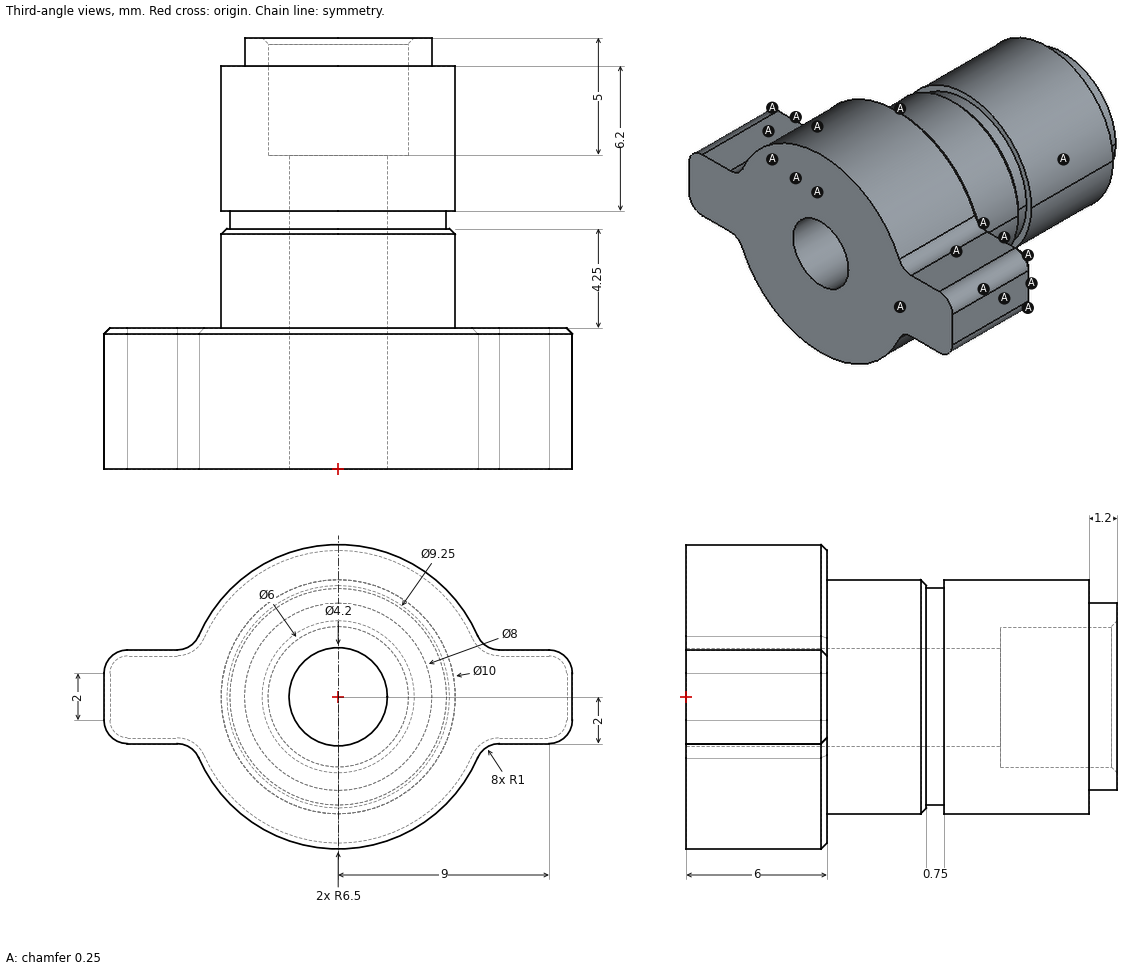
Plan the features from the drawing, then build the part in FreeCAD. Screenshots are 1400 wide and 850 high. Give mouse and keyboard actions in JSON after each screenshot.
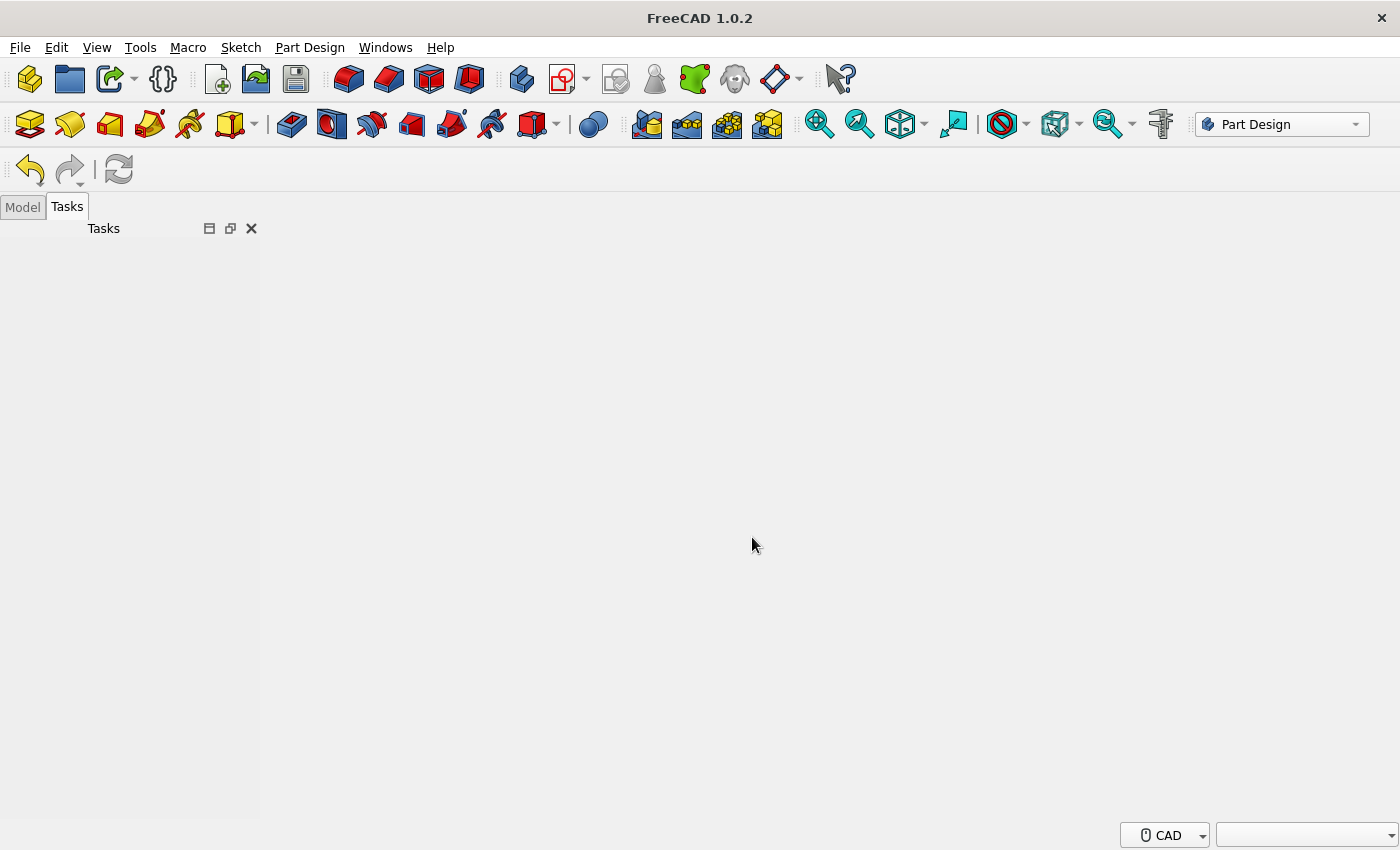
{"action": "left_click", "coordinate": [216, 80]}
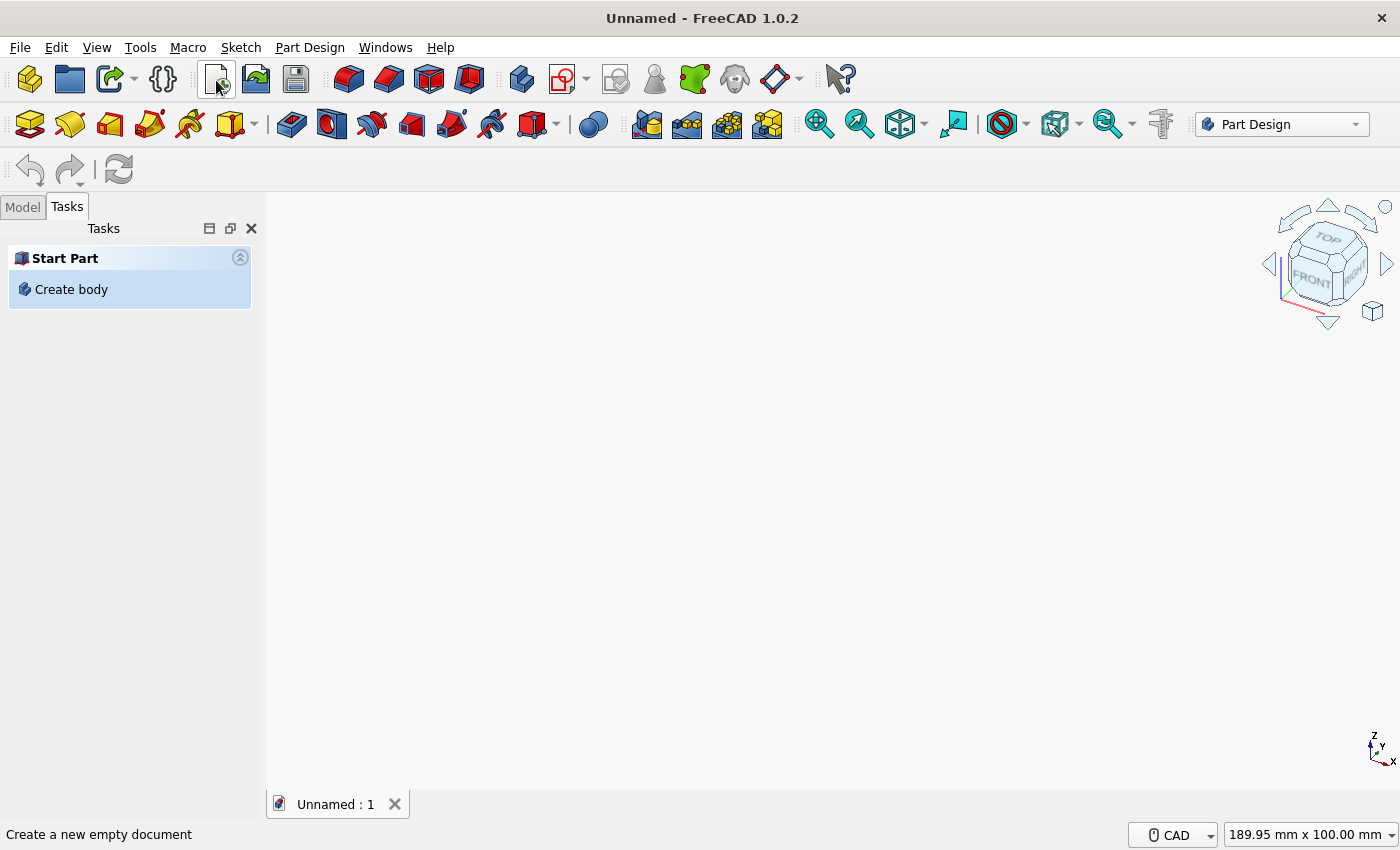
{"action": "left_click", "coordinate": [562, 80]}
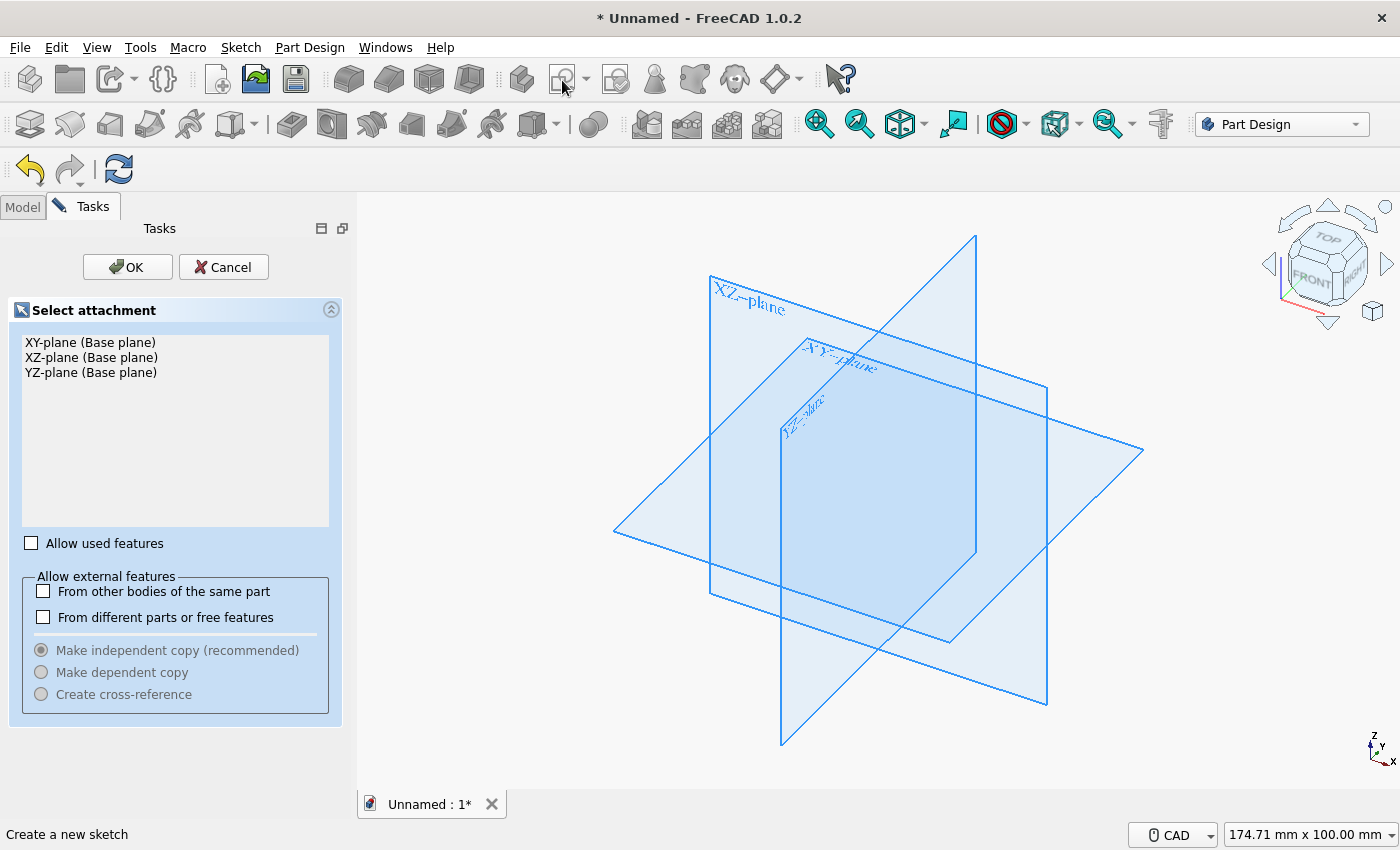
{"action": "left_click", "coordinate": [82, 358]}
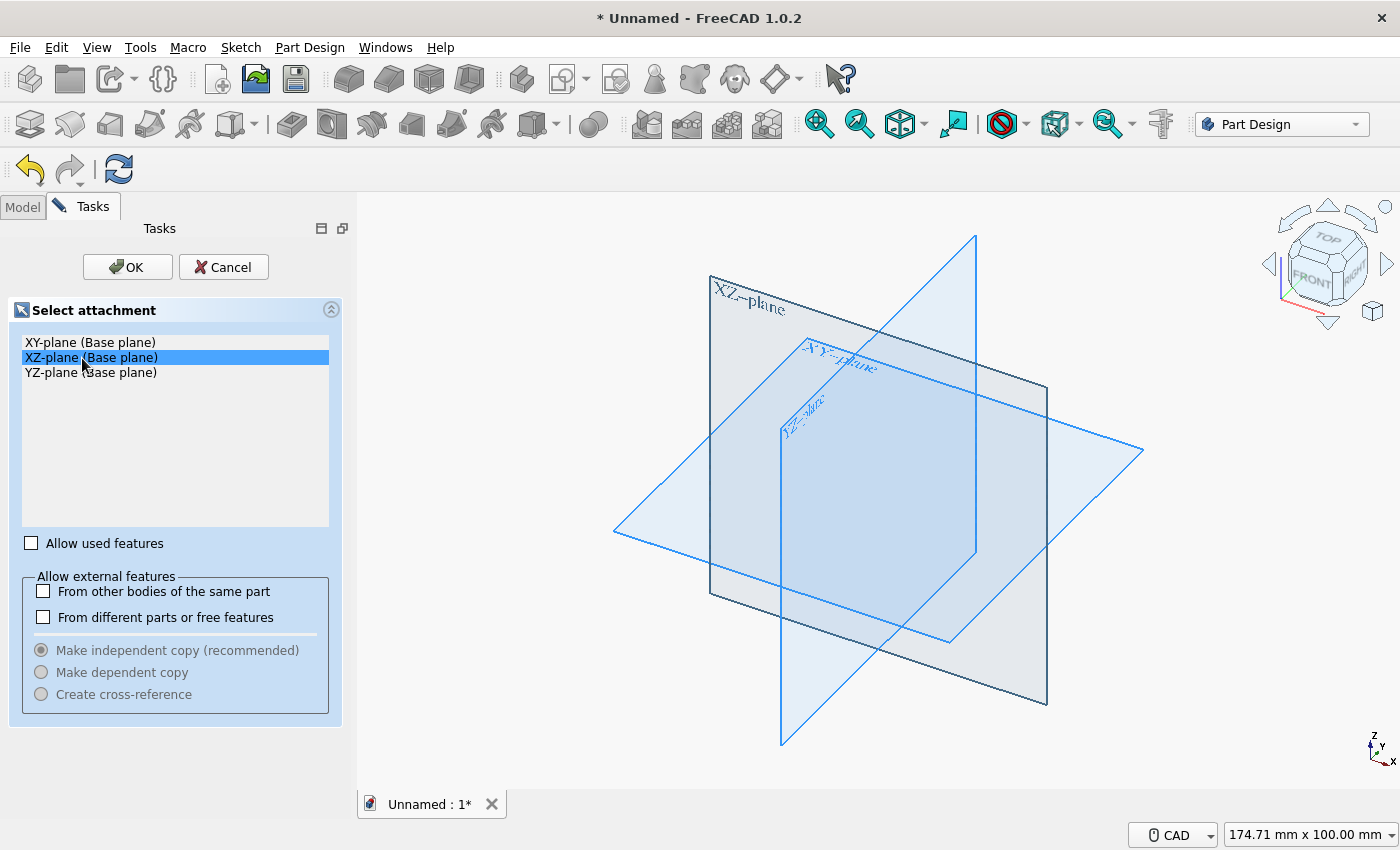
{"action": "left_click", "coordinate": [128, 267]}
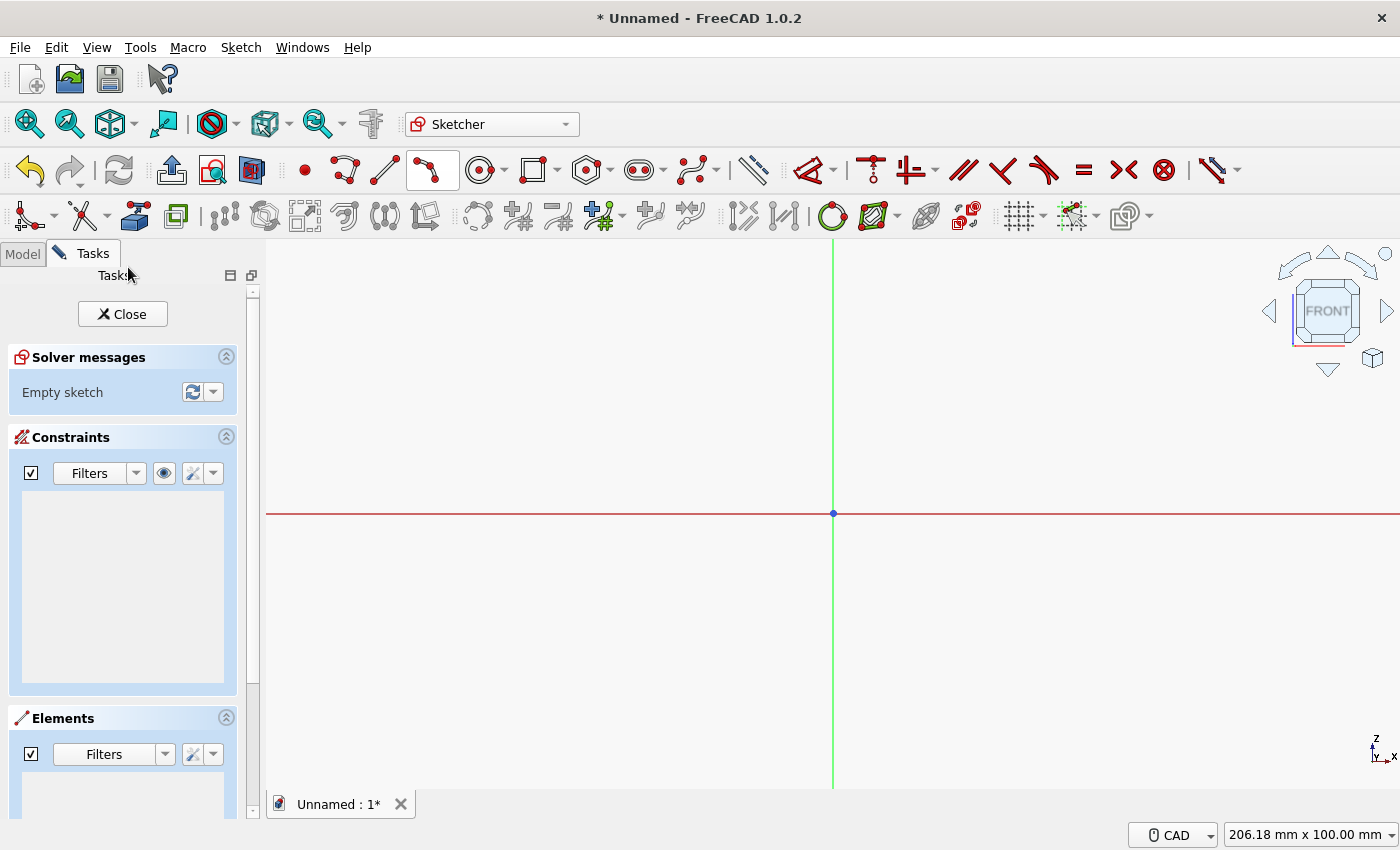
{"action": "scroll", "coordinate": [850, 514], "scroll_direction": "up", "scroll_amount": 8}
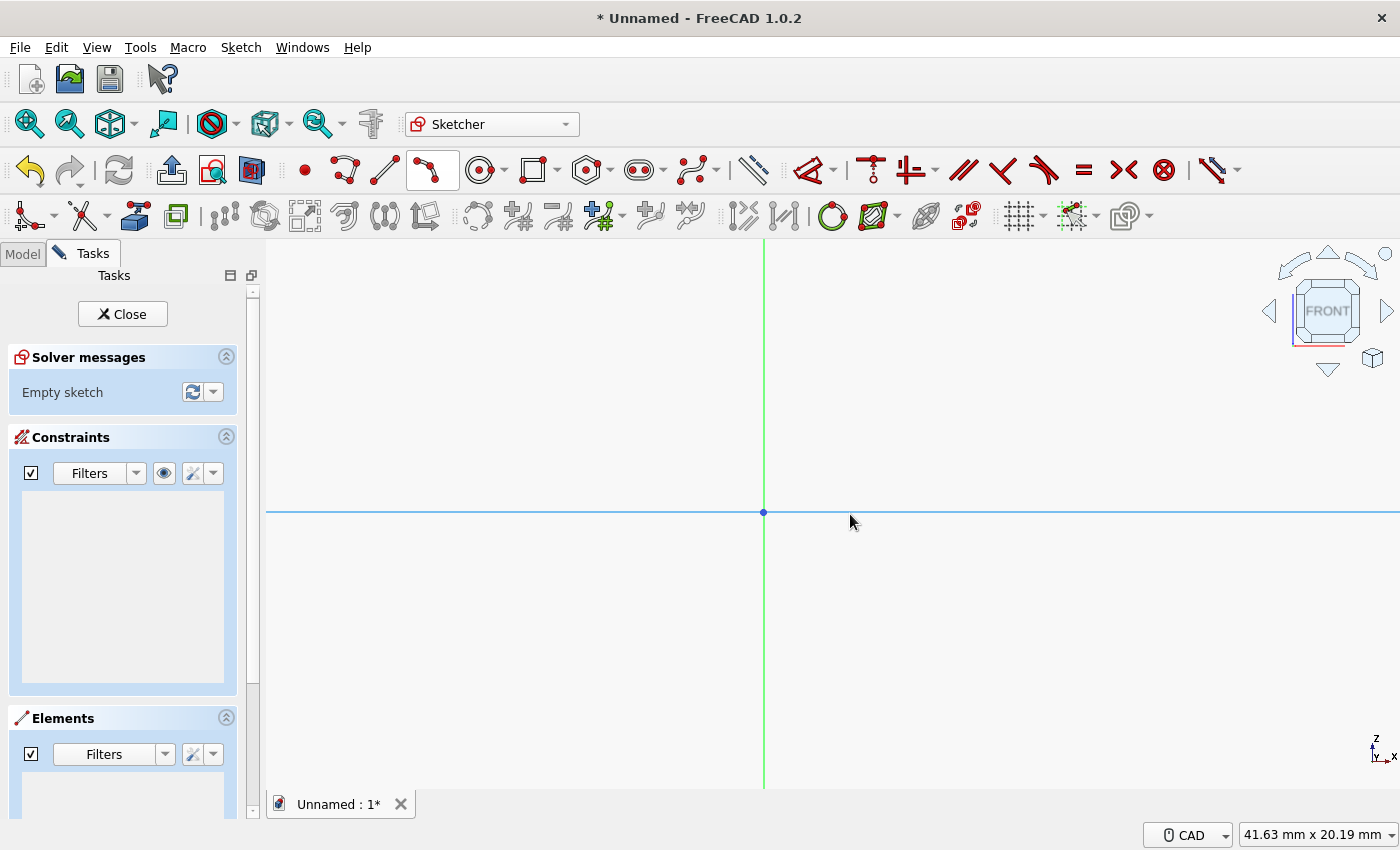
{"action": "left_click", "coordinate": [386, 170]}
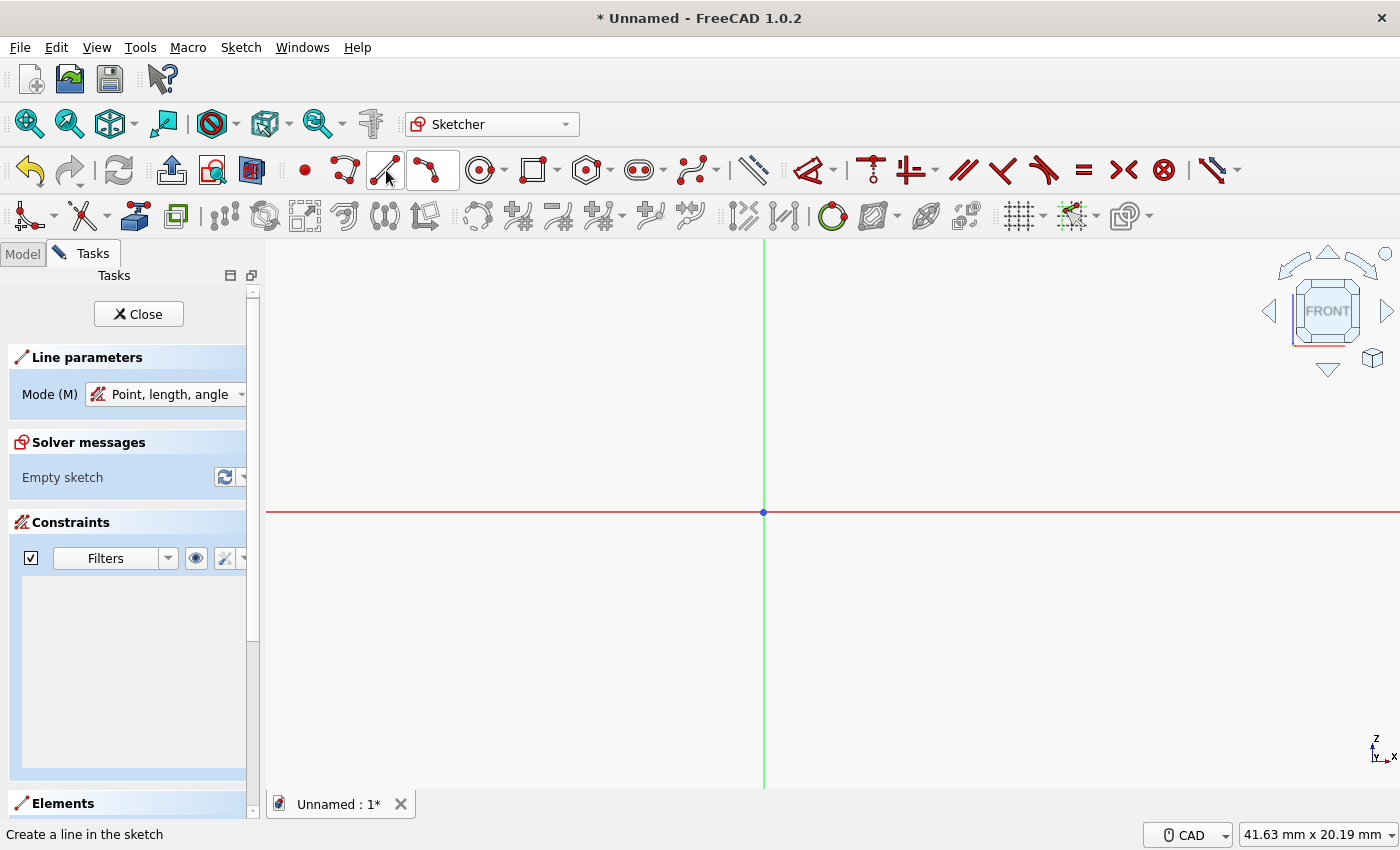
{"action": "left_click", "coordinate": [1009, 567]}
{"action": "left_click", "coordinate": [951, 567]}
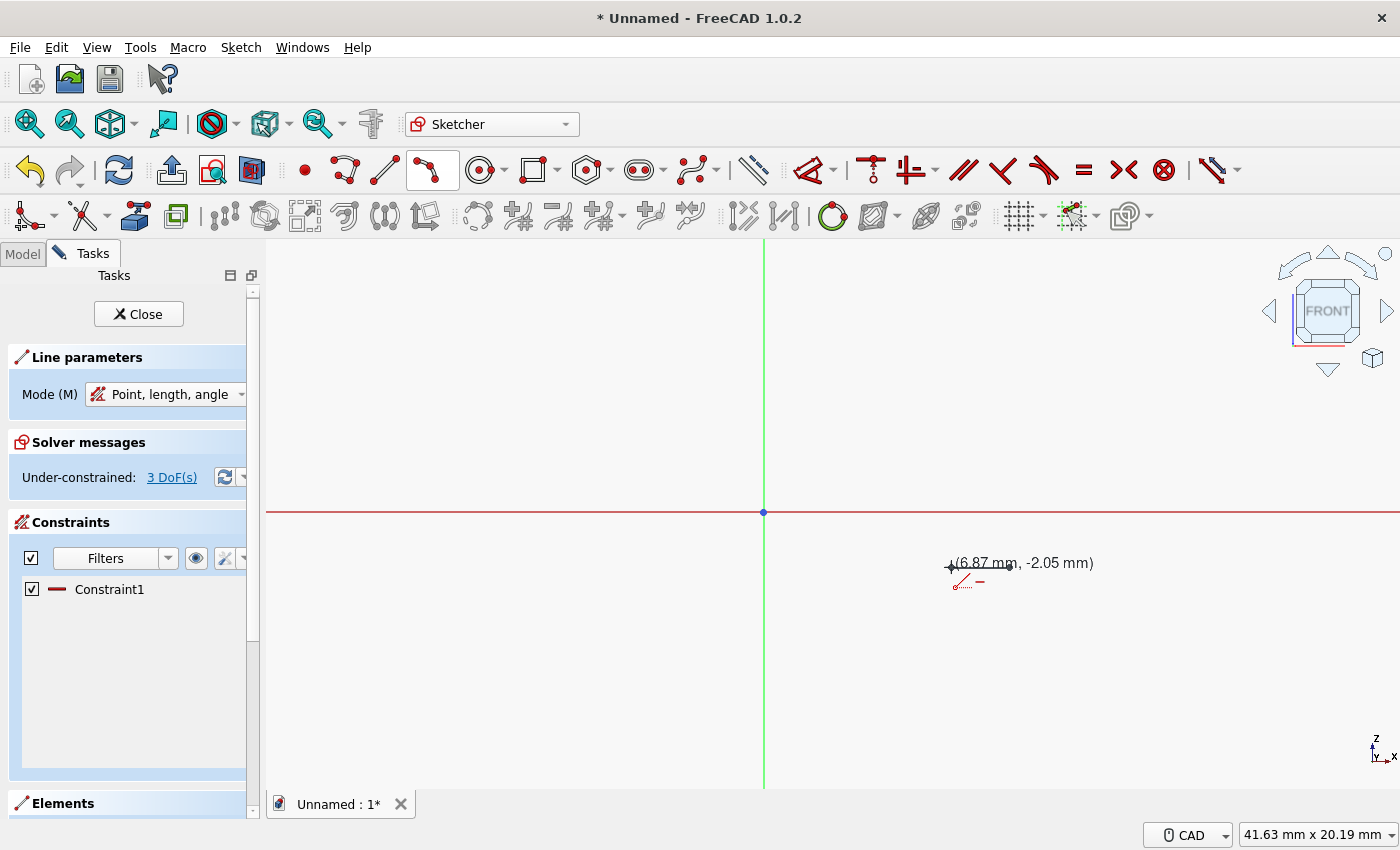
{"action": "left_click", "coordinate": [577, 567]}
{"action": "left_click", "coordinate": [519, 567]}